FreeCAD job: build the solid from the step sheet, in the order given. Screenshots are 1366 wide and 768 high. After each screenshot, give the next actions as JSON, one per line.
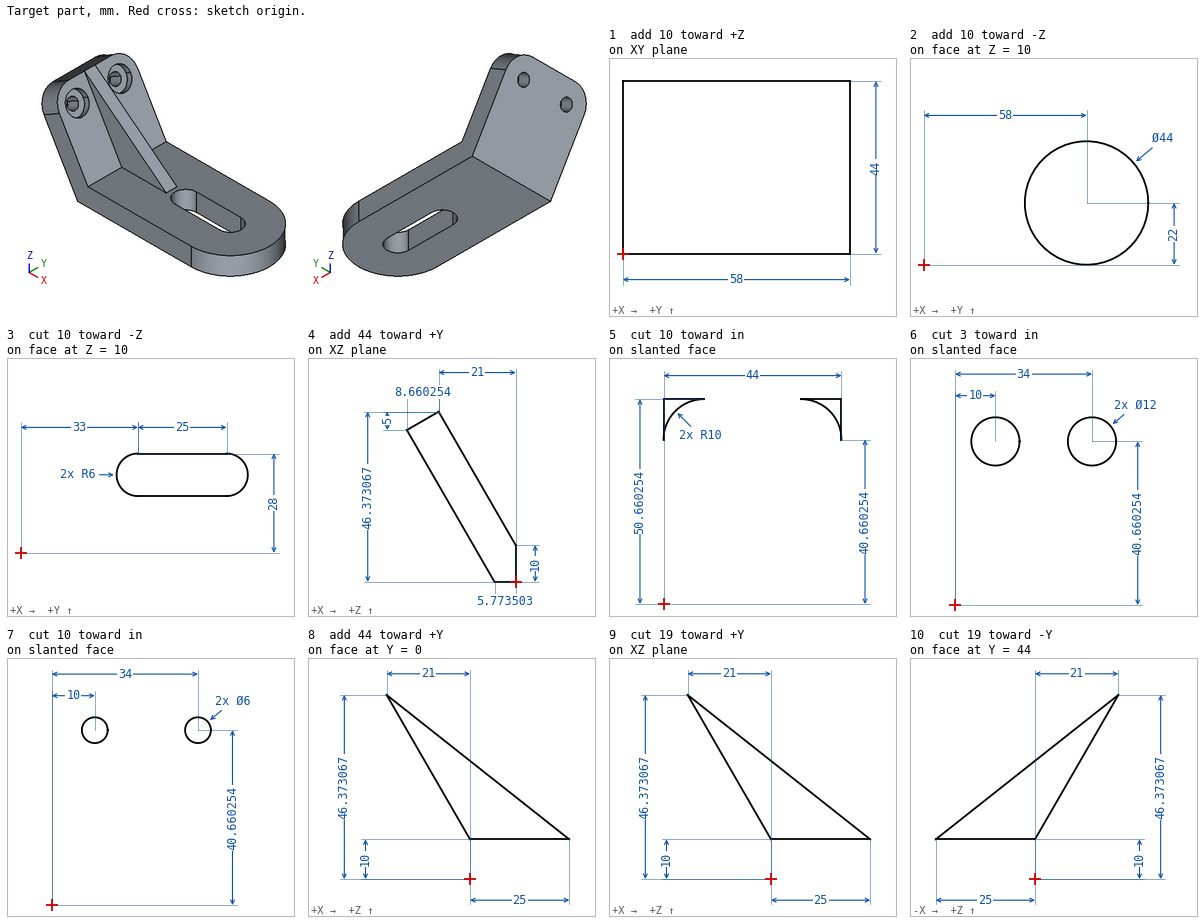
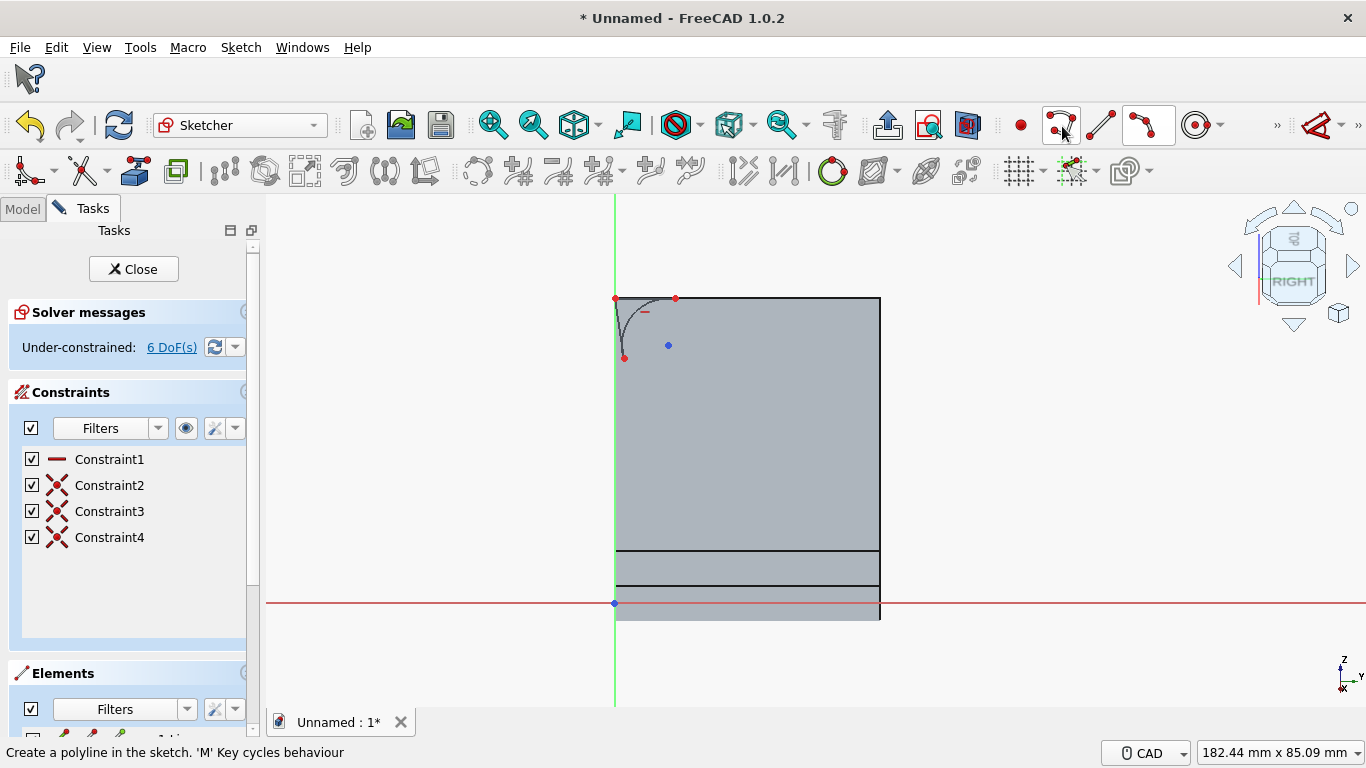
{"action": "left_click", "coordinate": [880, 358]}
{"action": "left_click", "coordinate": [880, 298]}
{"action": "left_click", "coordinate": [820, 298]}
{"action": "right_click", "coordinate": [820, 298]}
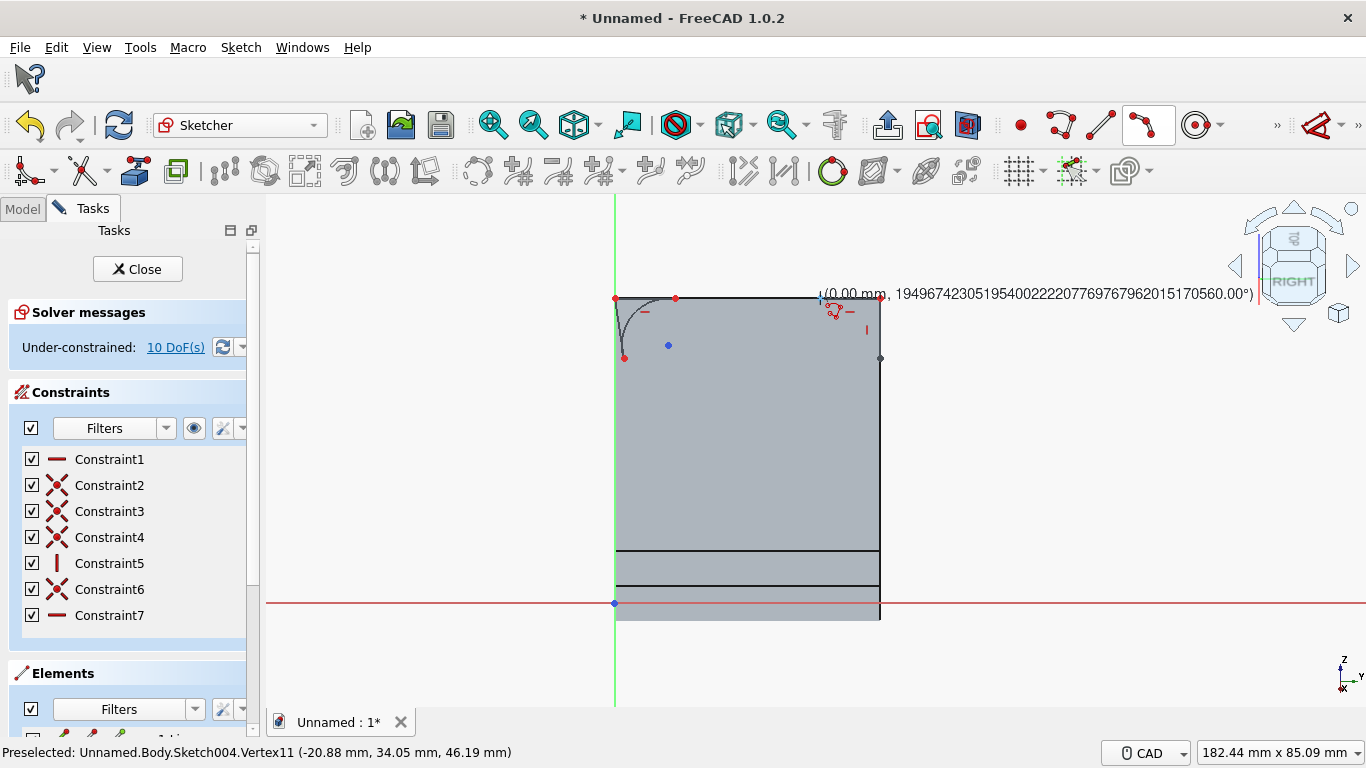
{"action": "key", "text": "g 3 a"}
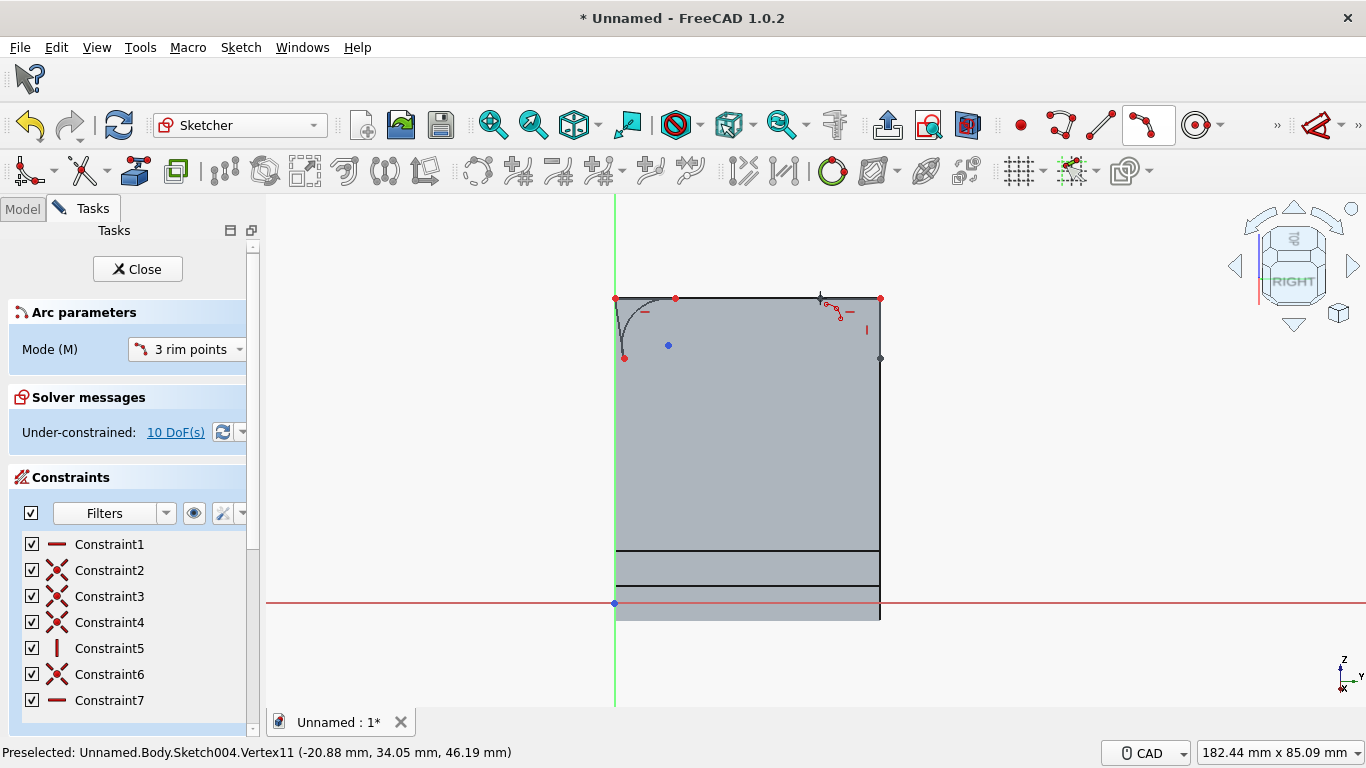
{"action": "left_click", "coordinate": [820, 299]}
{"action": "left_click", "coordinate": [880, 359]}
{"action": "left_click", "coordinate": [862, 315]}
{"action": "key", "text": "Escape"}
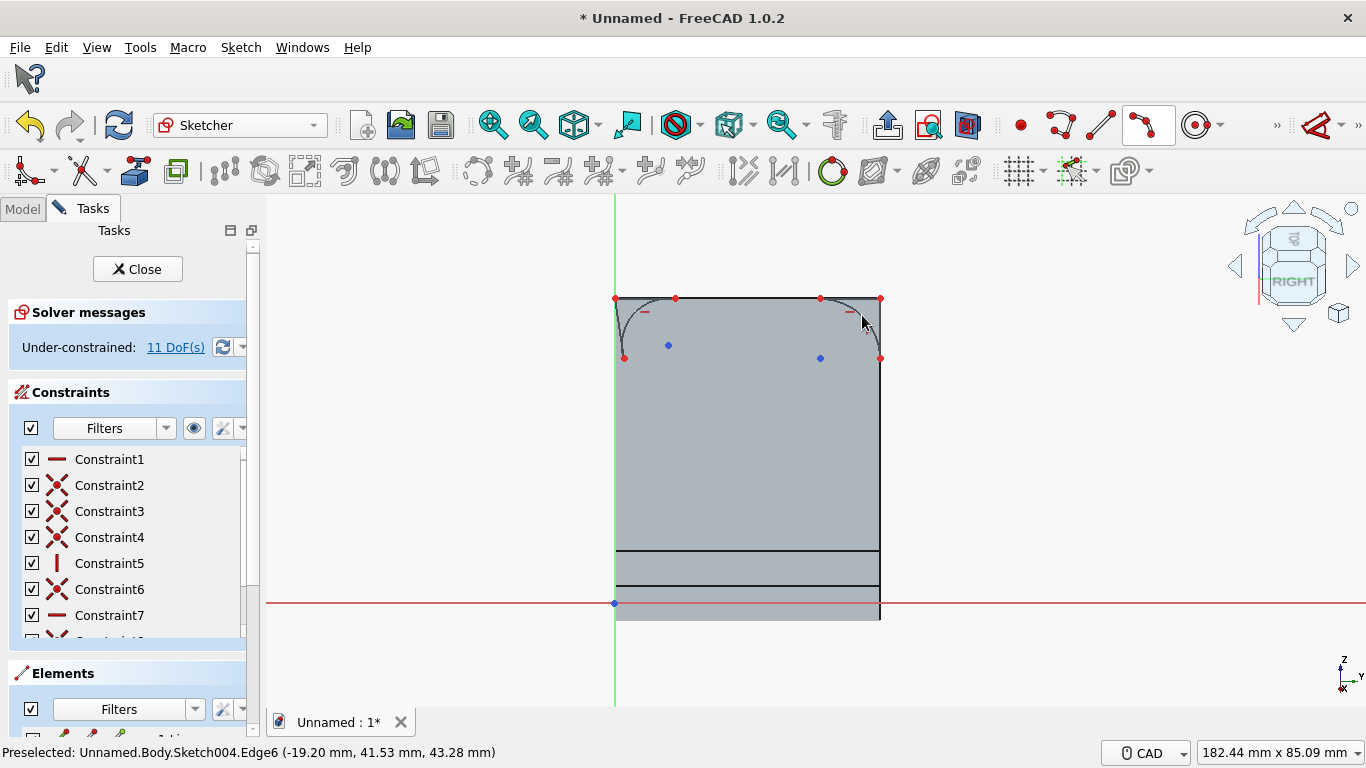
{"action": "left_click", "coordinate": [633, 299]}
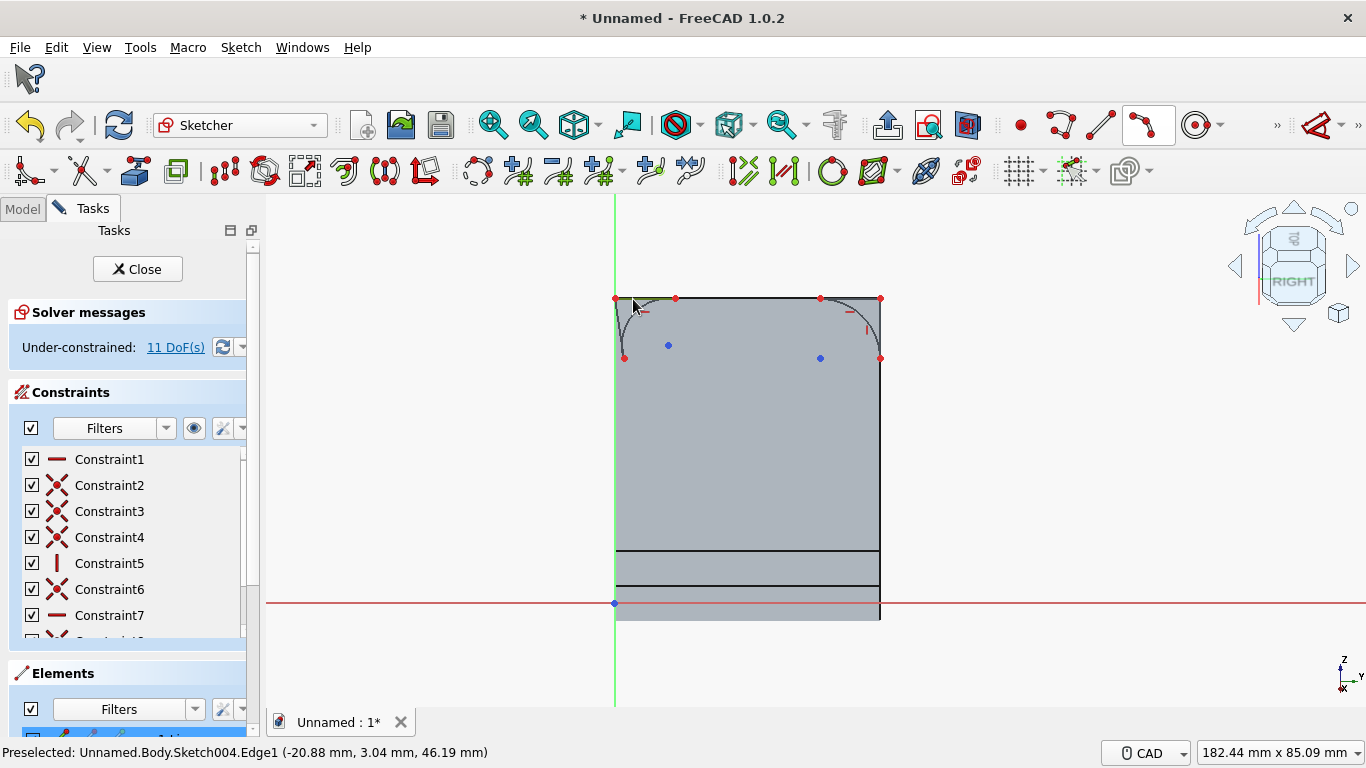
{"action": "left_click", "coordinate": [633, 315]}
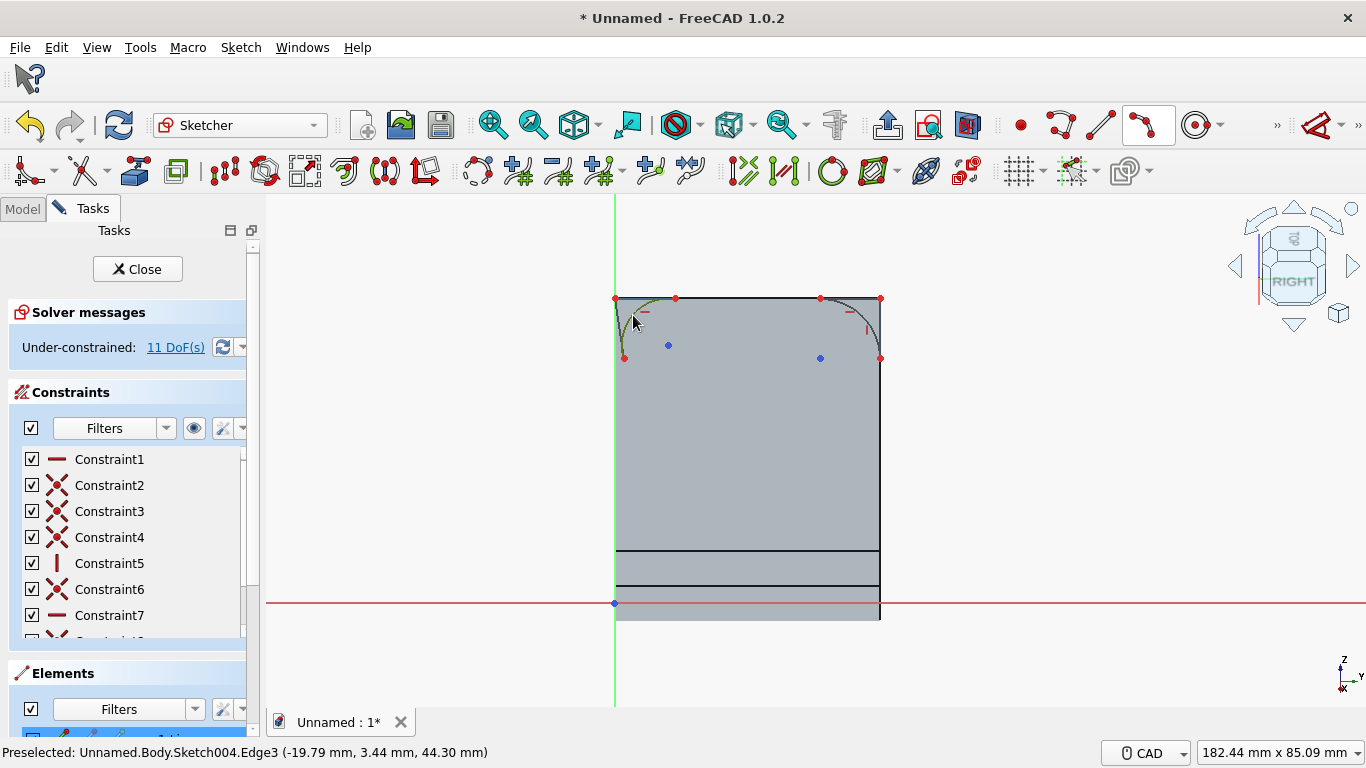
{"action": "key", "text": "t"}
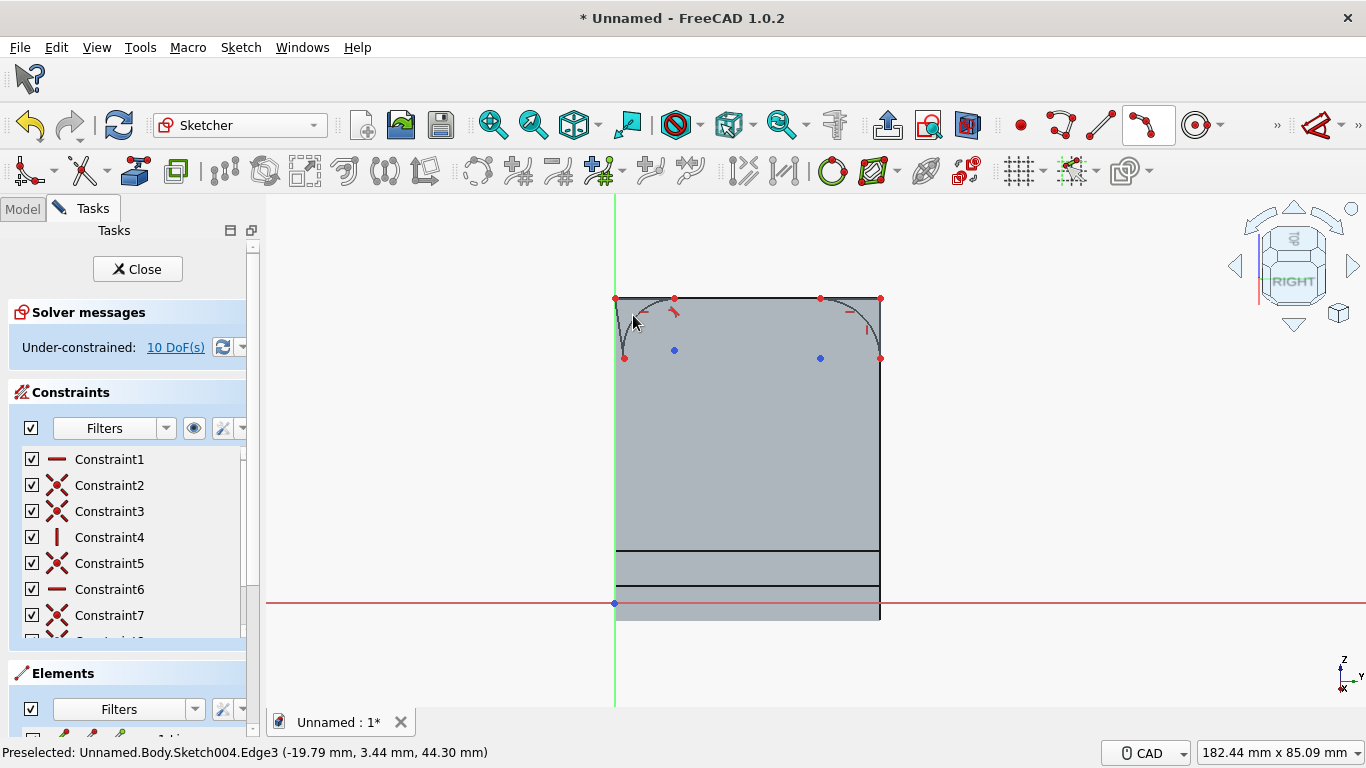
{"action": "left_click", "coordinate": [618, 317]}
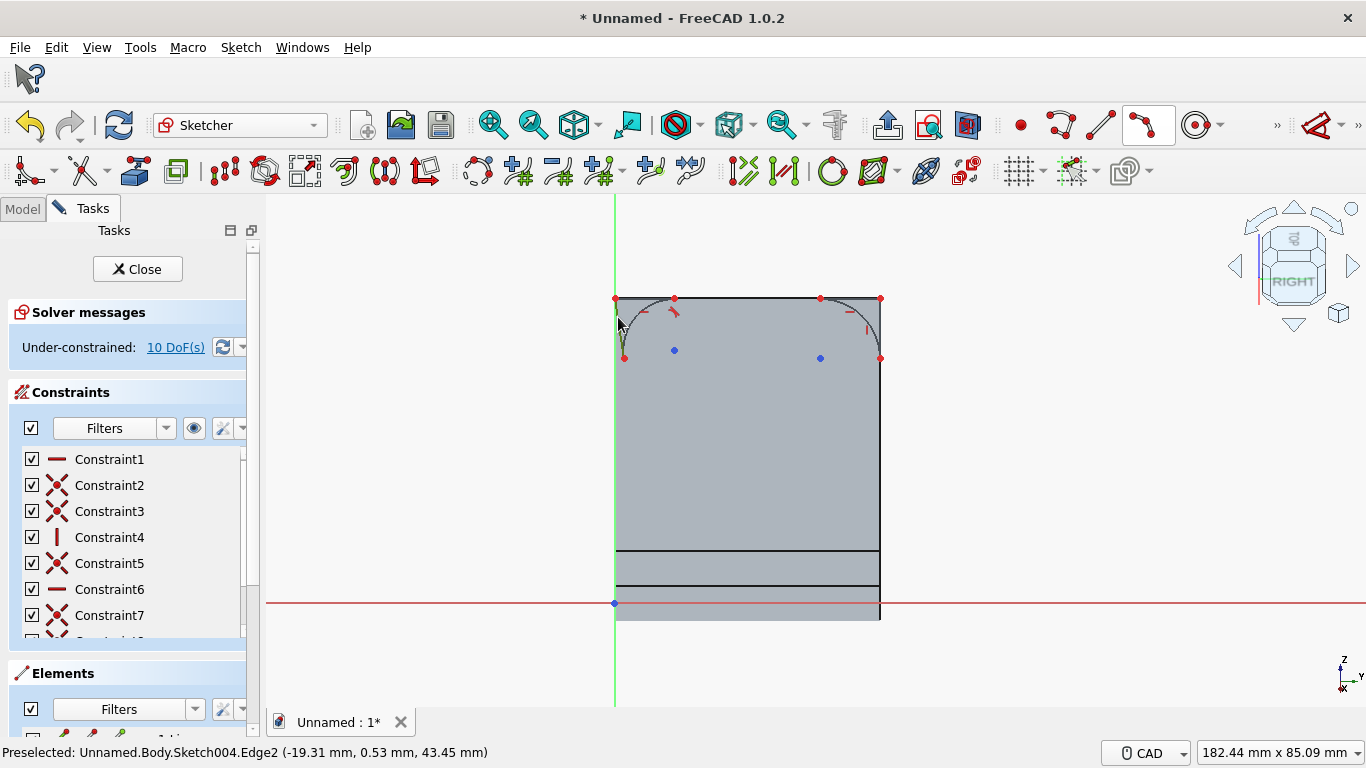
{"action": "left_click", "coordinate": [636, 317]}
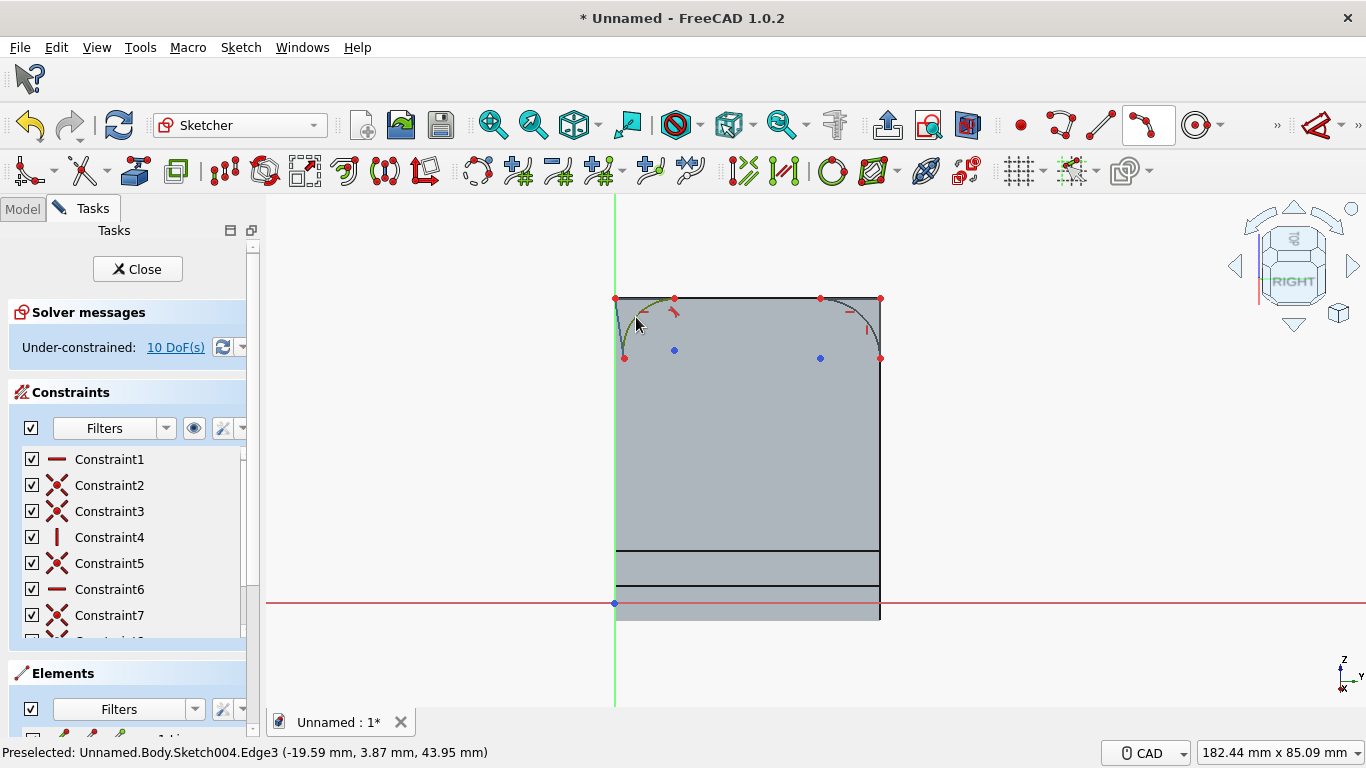
{"action": "key", "text": "t"}